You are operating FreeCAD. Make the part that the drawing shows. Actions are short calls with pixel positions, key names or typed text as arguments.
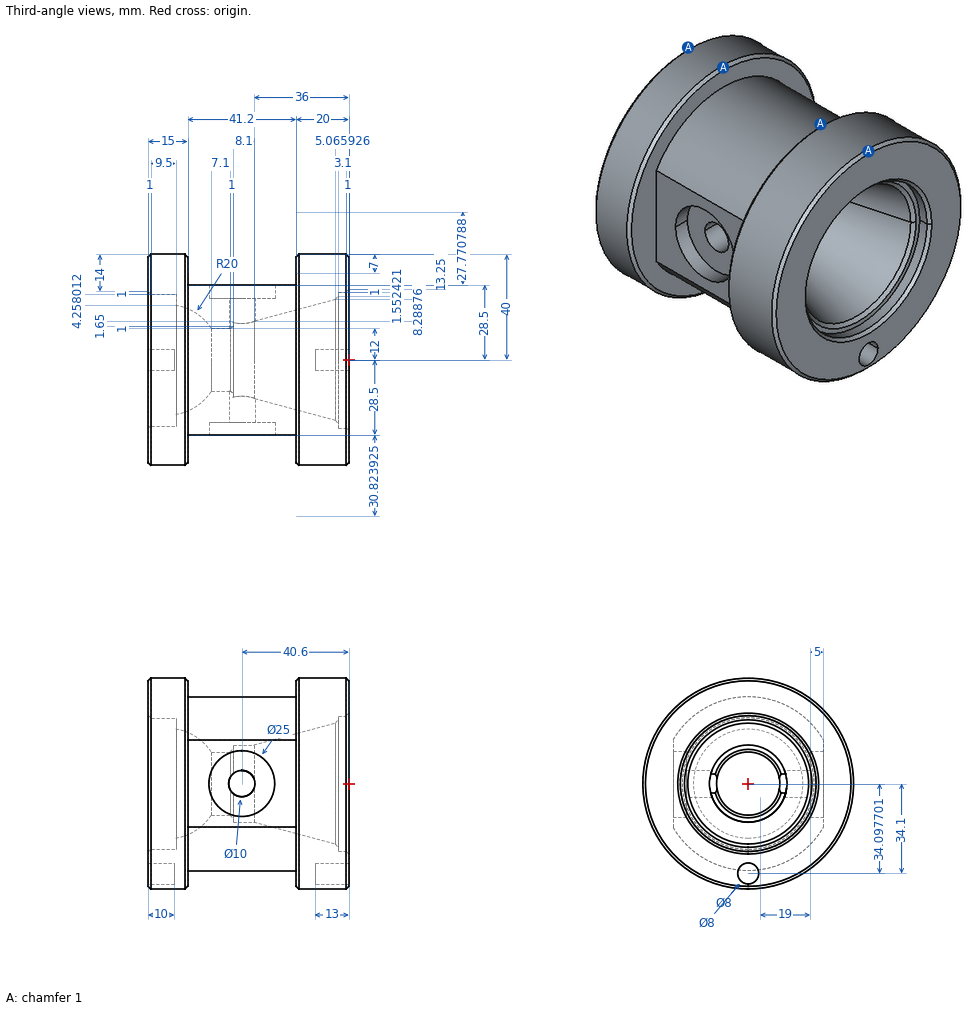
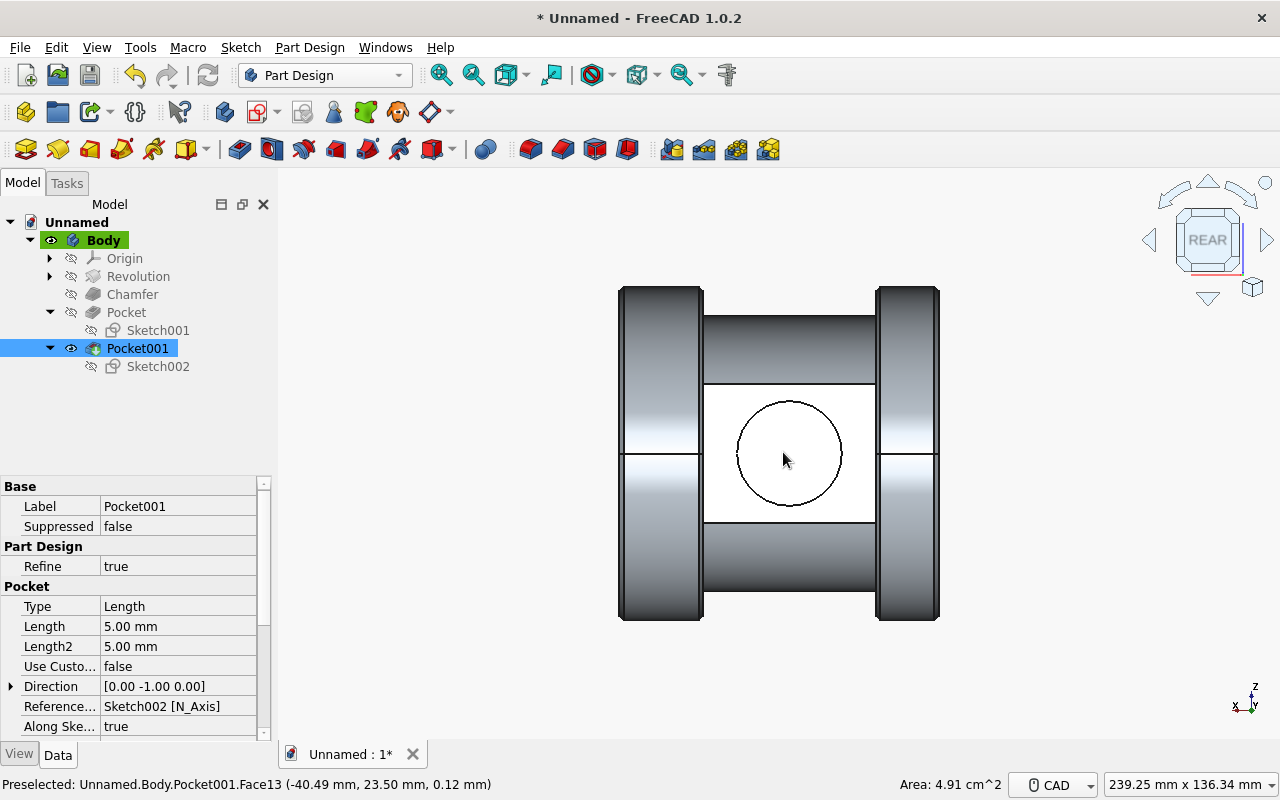
click(258, 112)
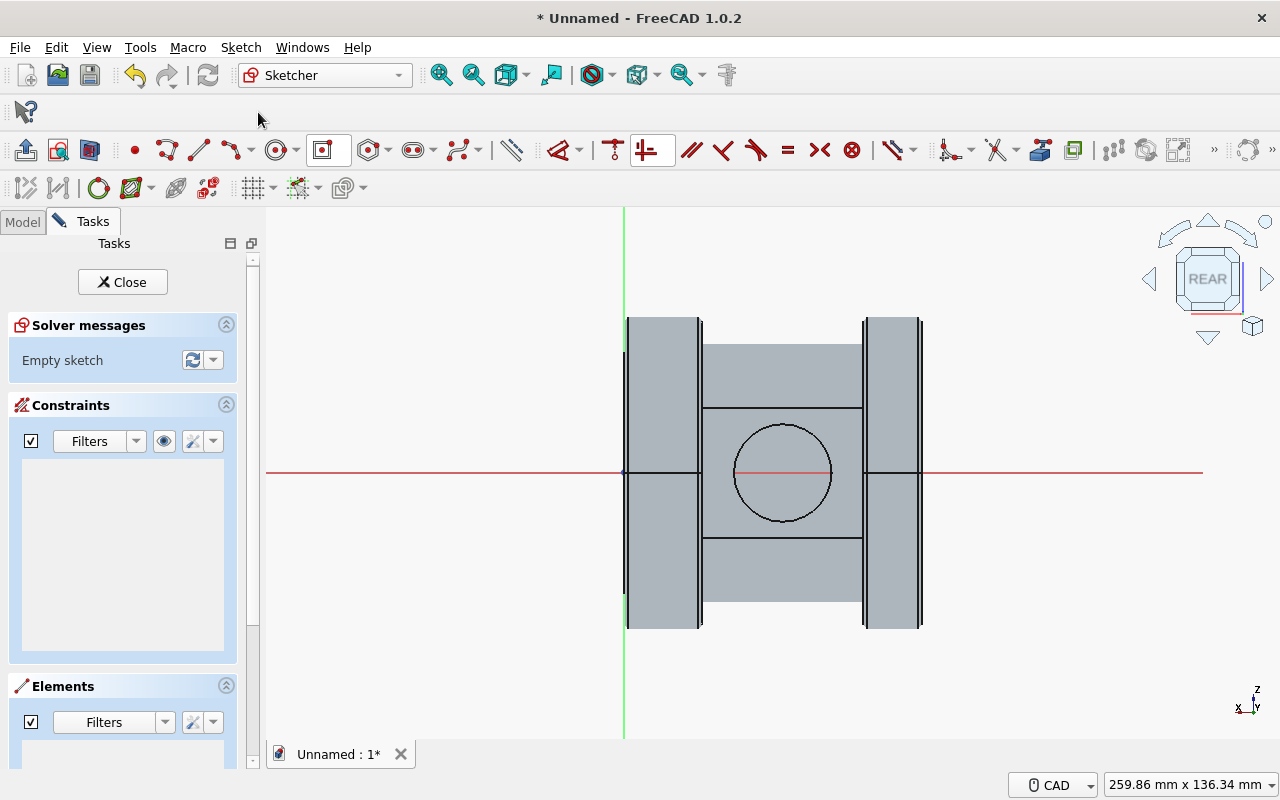
click(90, 150)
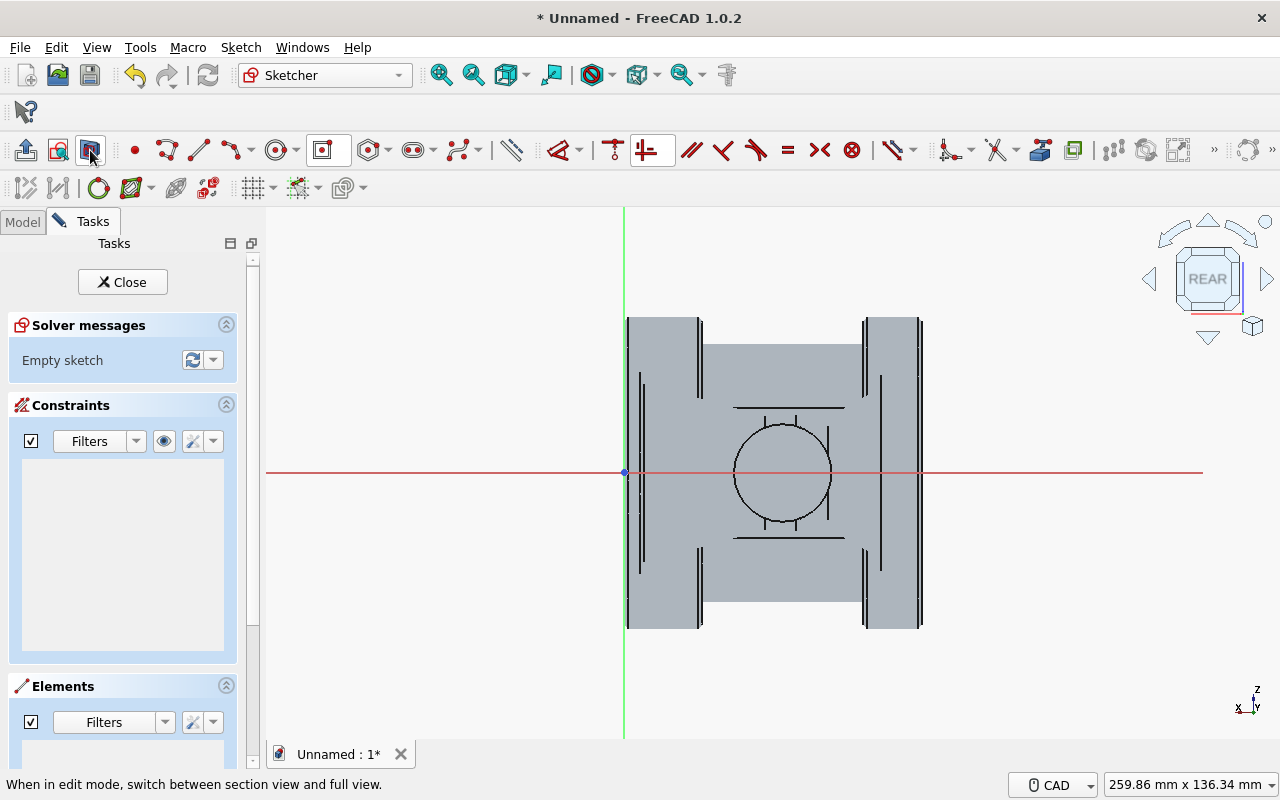
scroll(793, 473, up, 11)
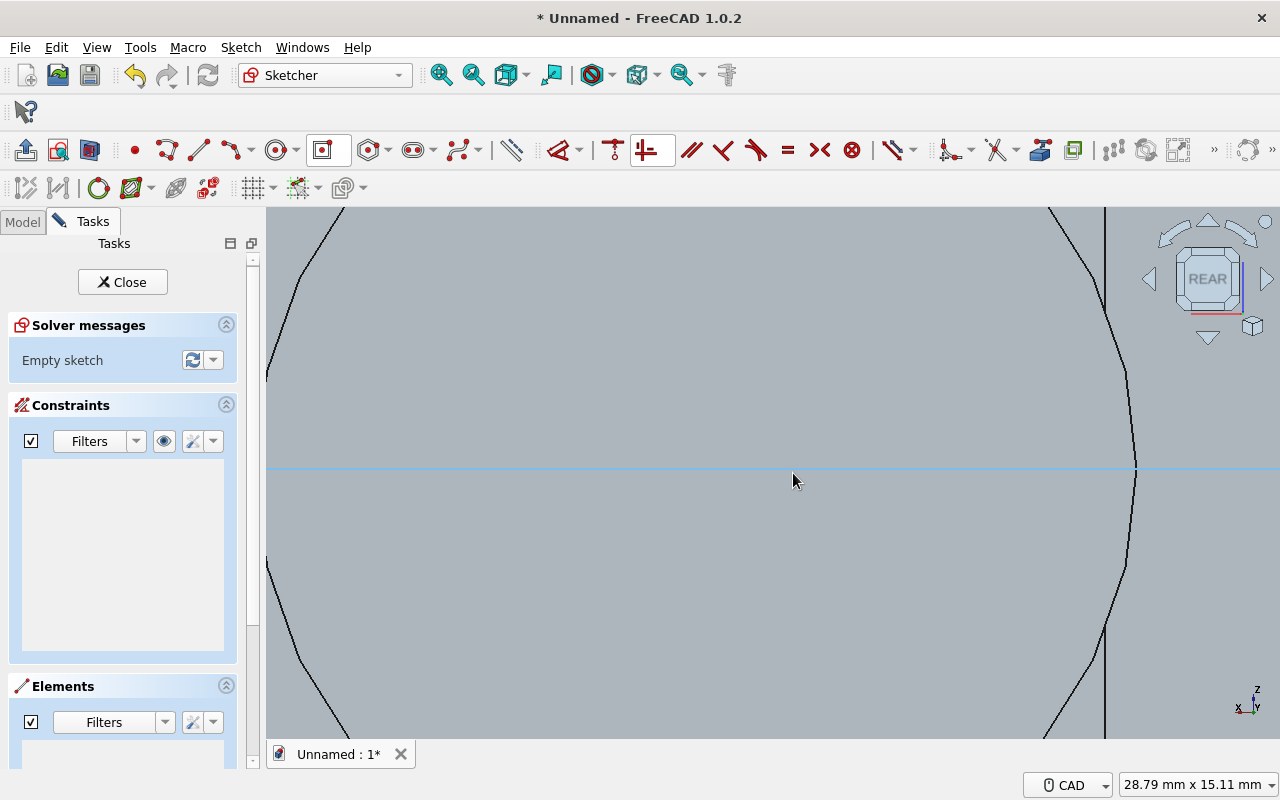
key(g)
key(c)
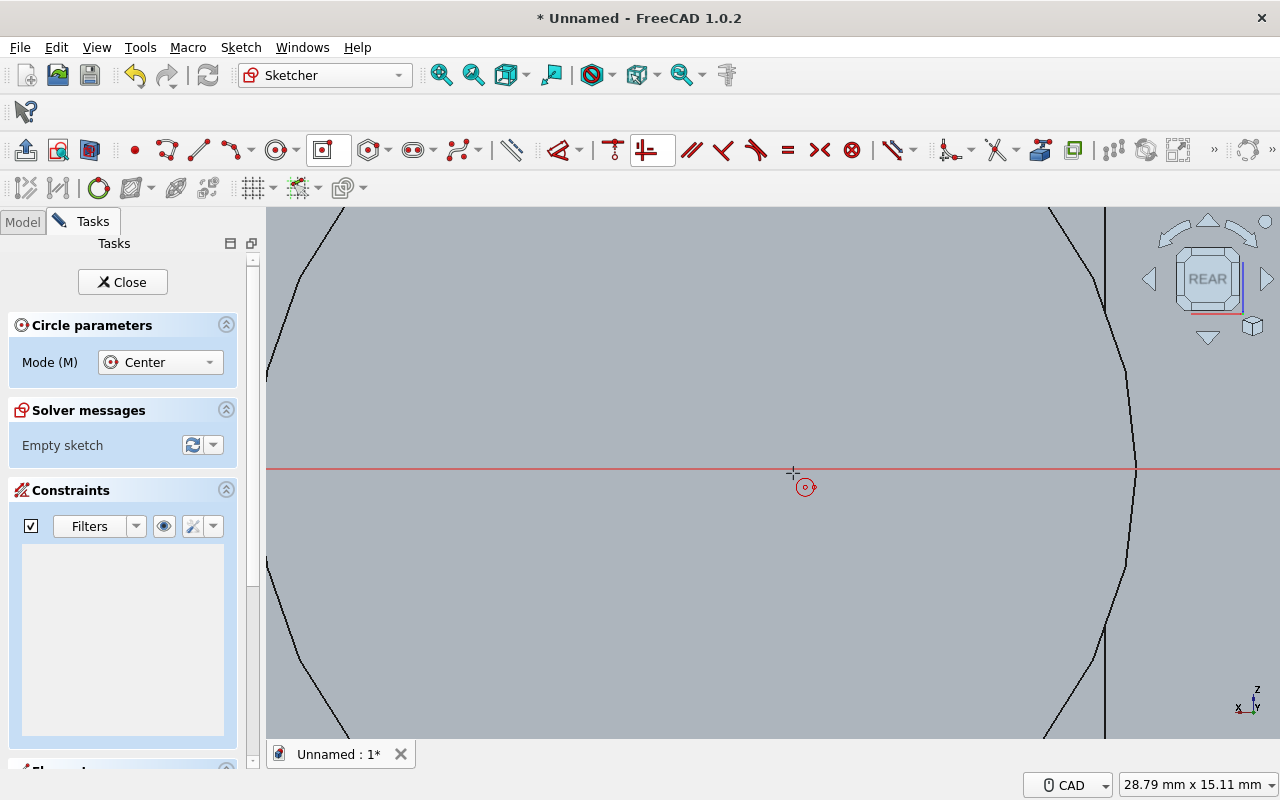
click(696, 469)
move(821, 344)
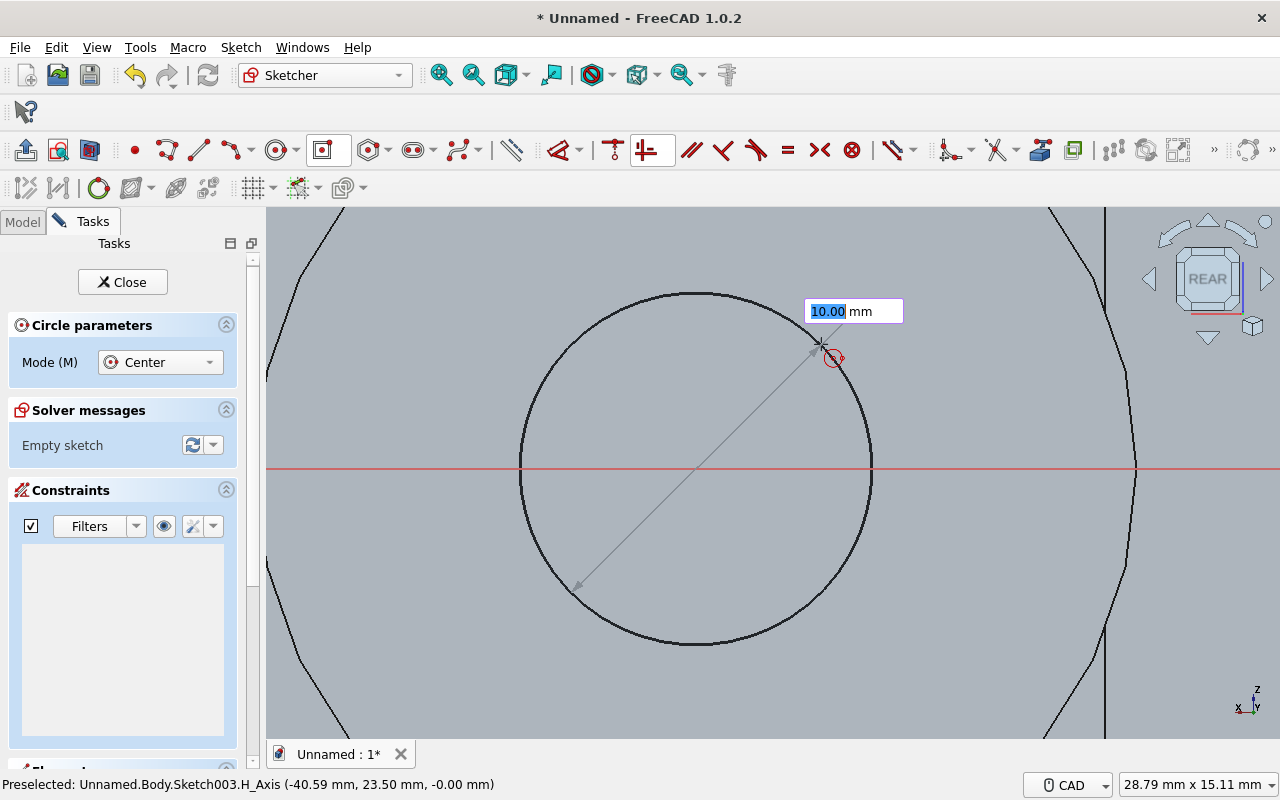
text(10)
key(Return)
key(Escape)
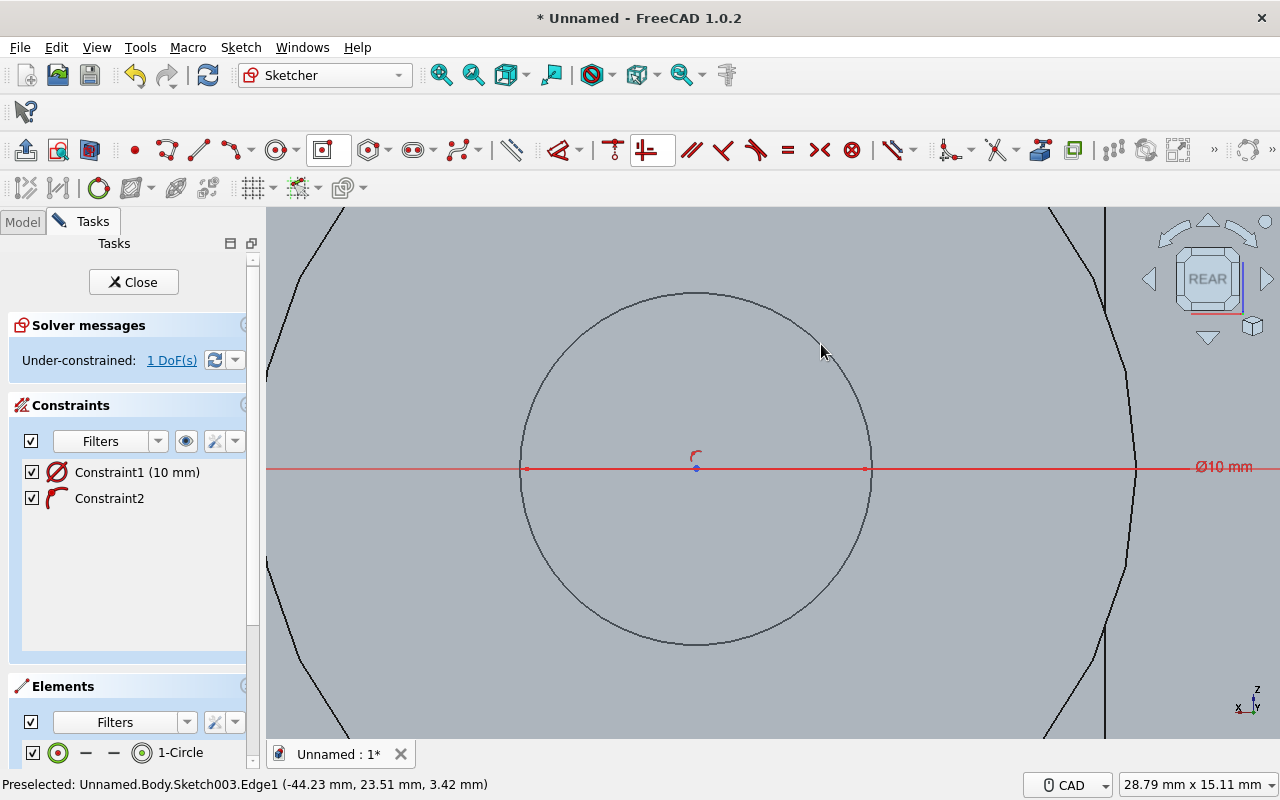
click(558, 150)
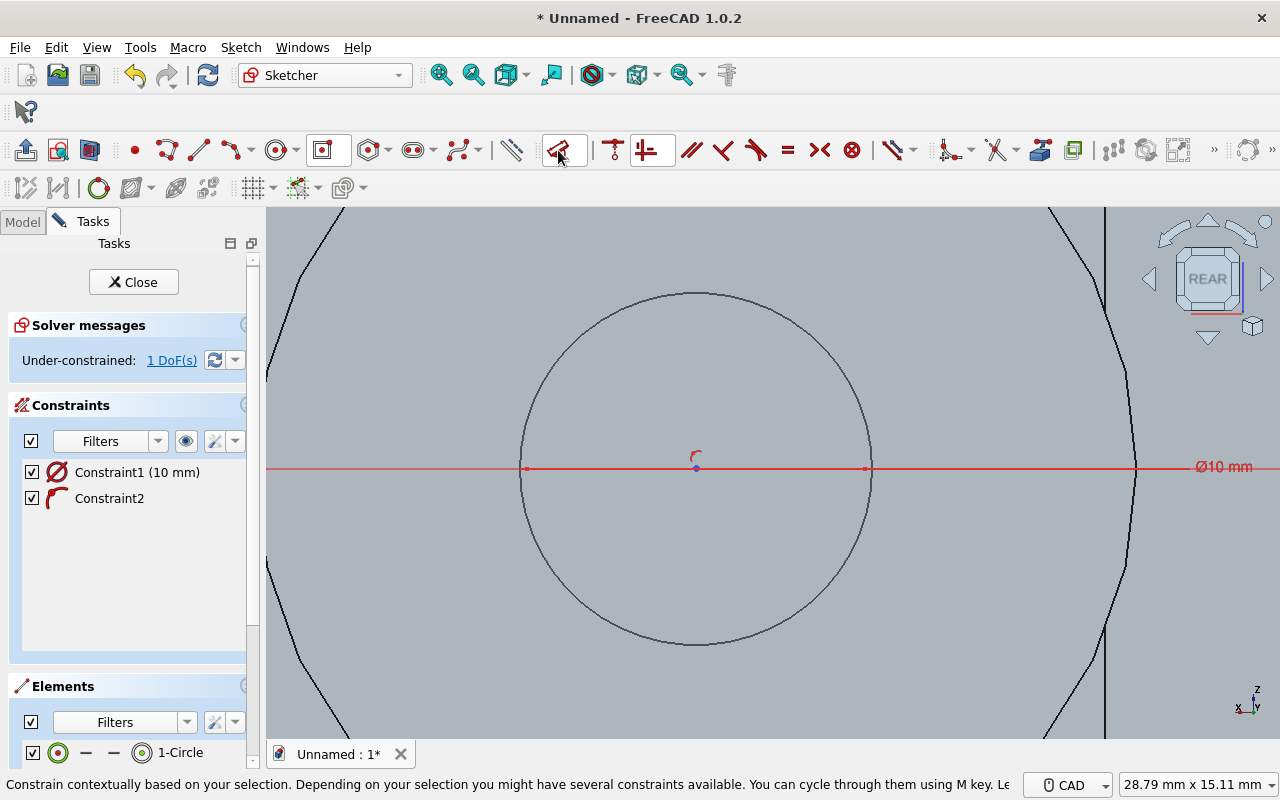
click(696, 469)
click(495, 503)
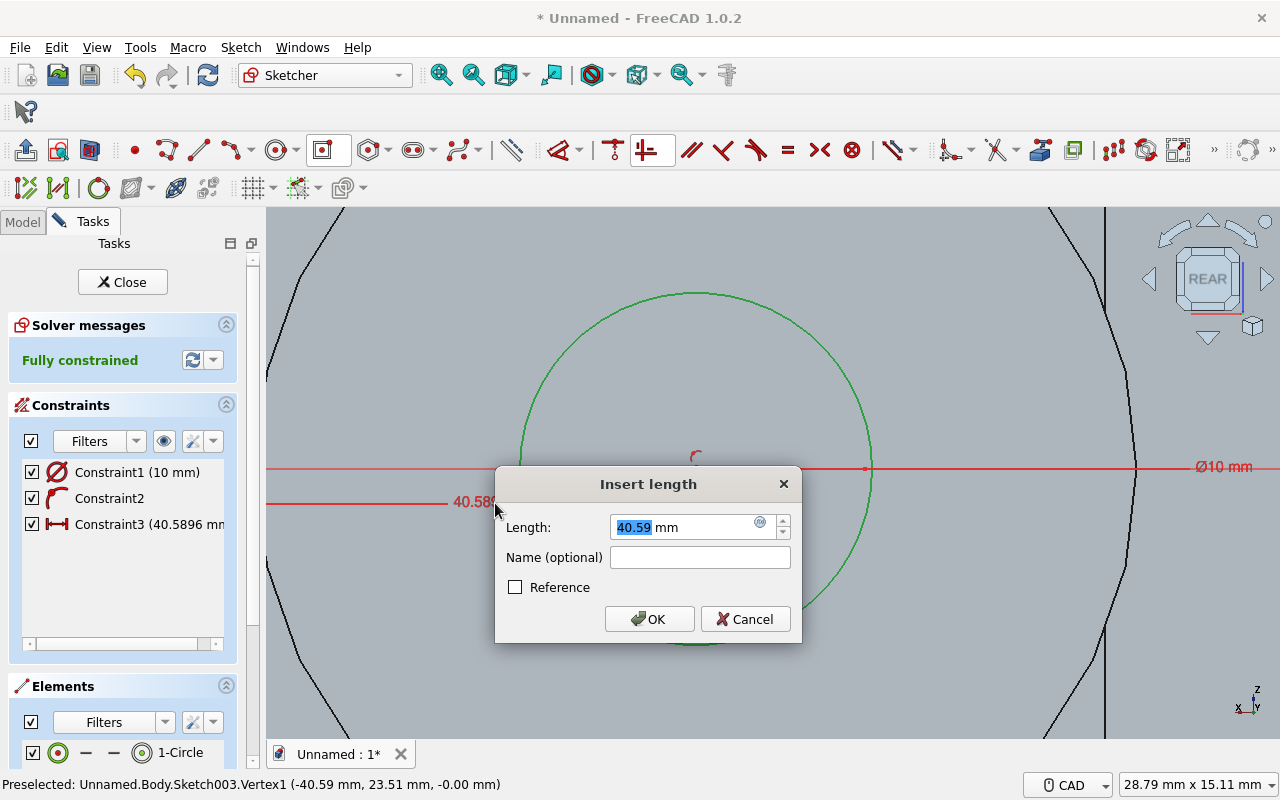
text(40.6)
key(Return)
key(Escape)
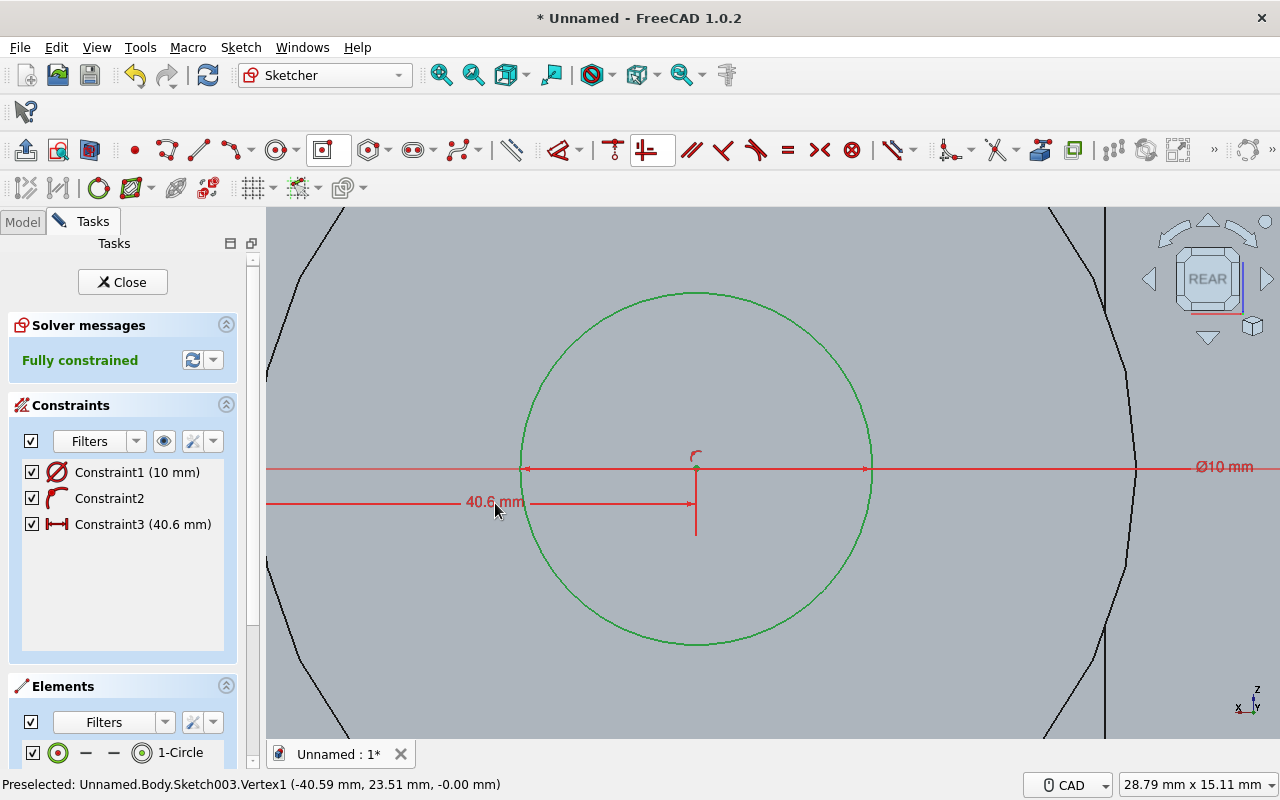
click(123, 282)